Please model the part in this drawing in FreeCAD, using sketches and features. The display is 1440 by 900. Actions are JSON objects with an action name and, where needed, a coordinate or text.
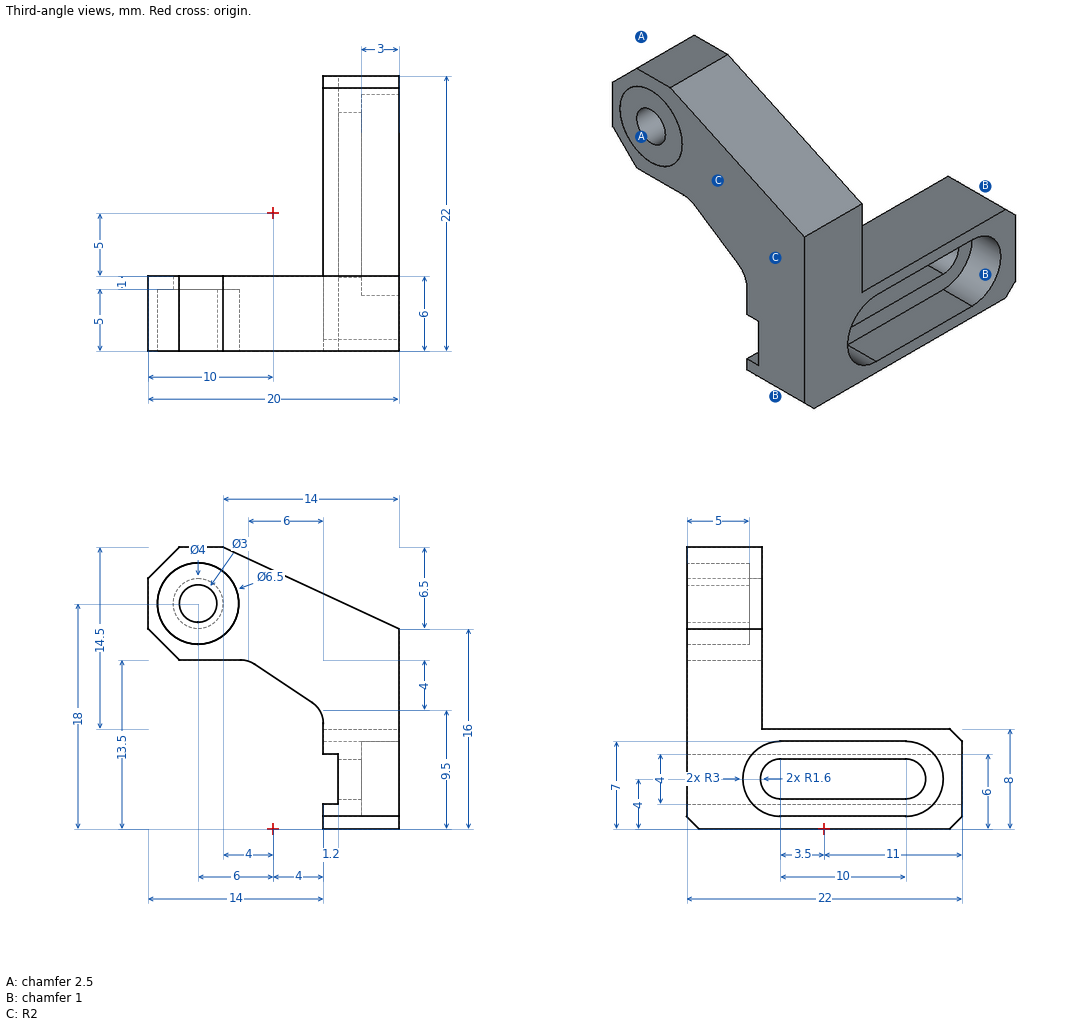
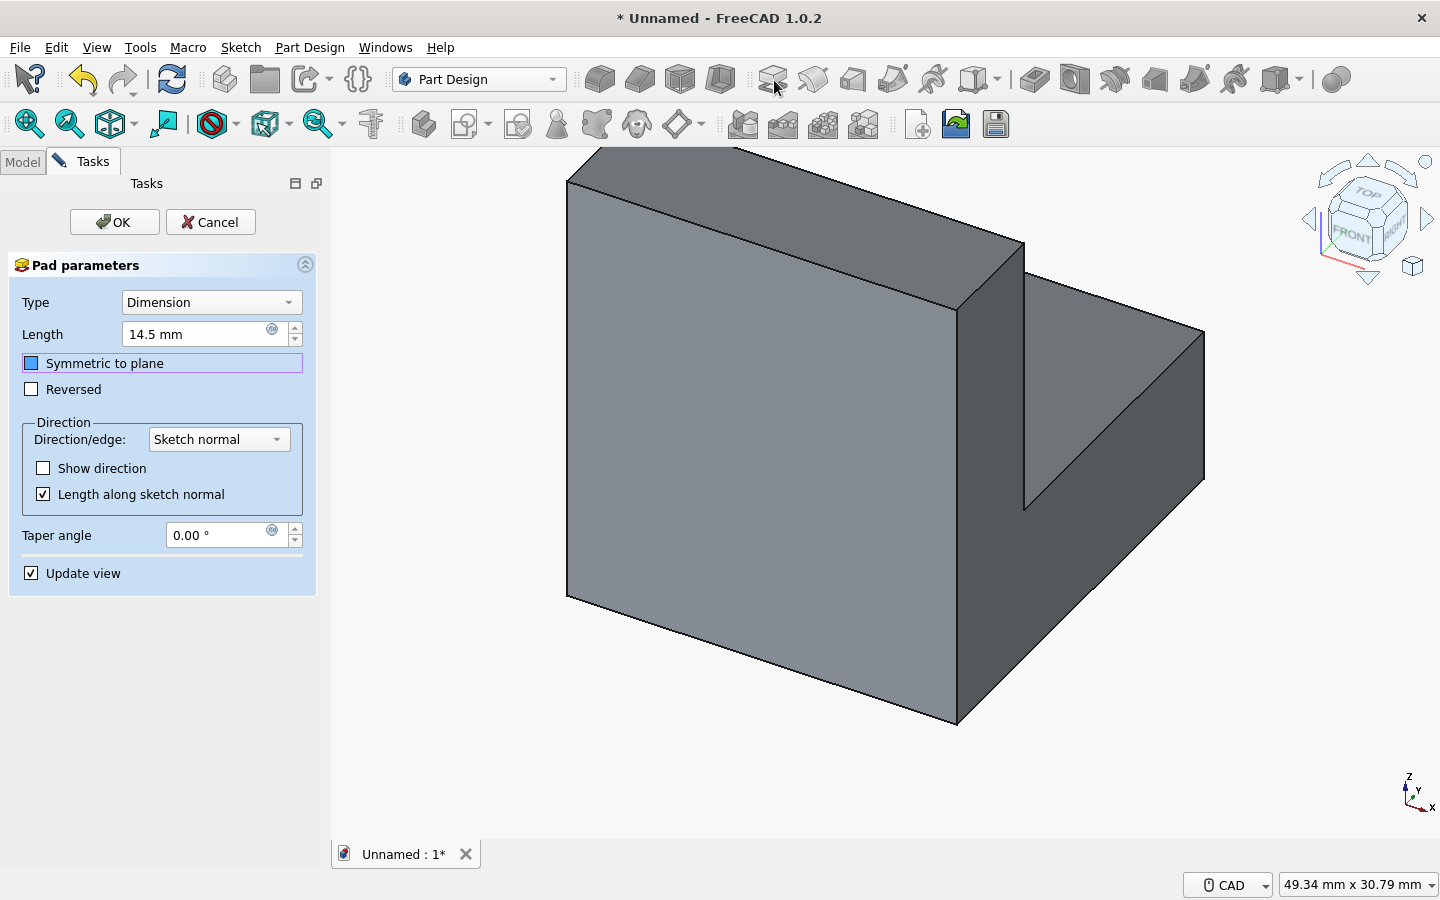
{"action": "left_click", "coordinate": [115, 222]}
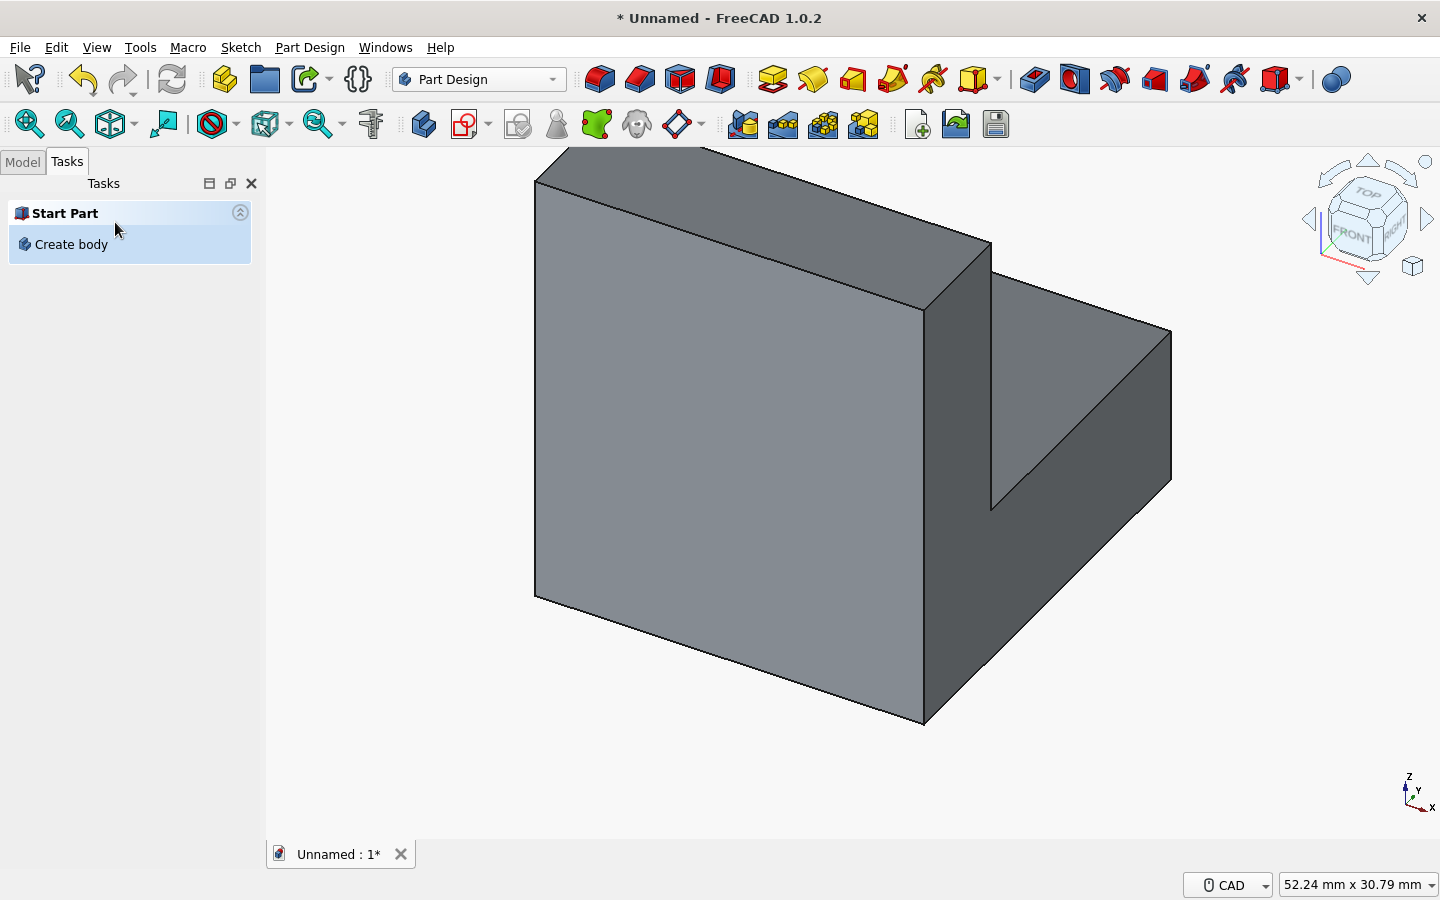
{"action": "left_click", "coordinate": [30, 124]}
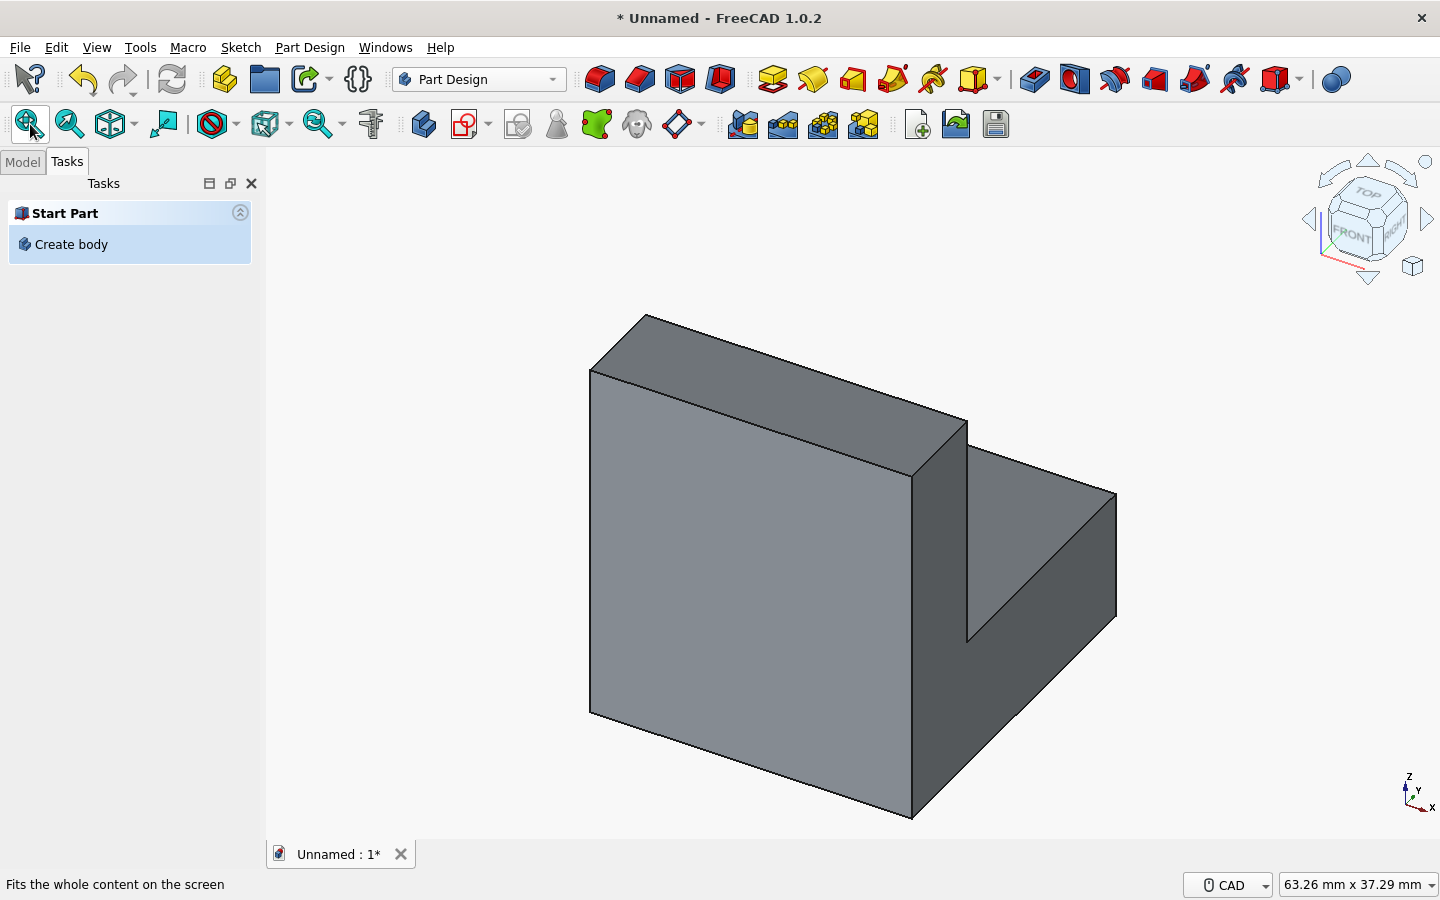
{"action": "left_click", "coordinate": [751, 593]}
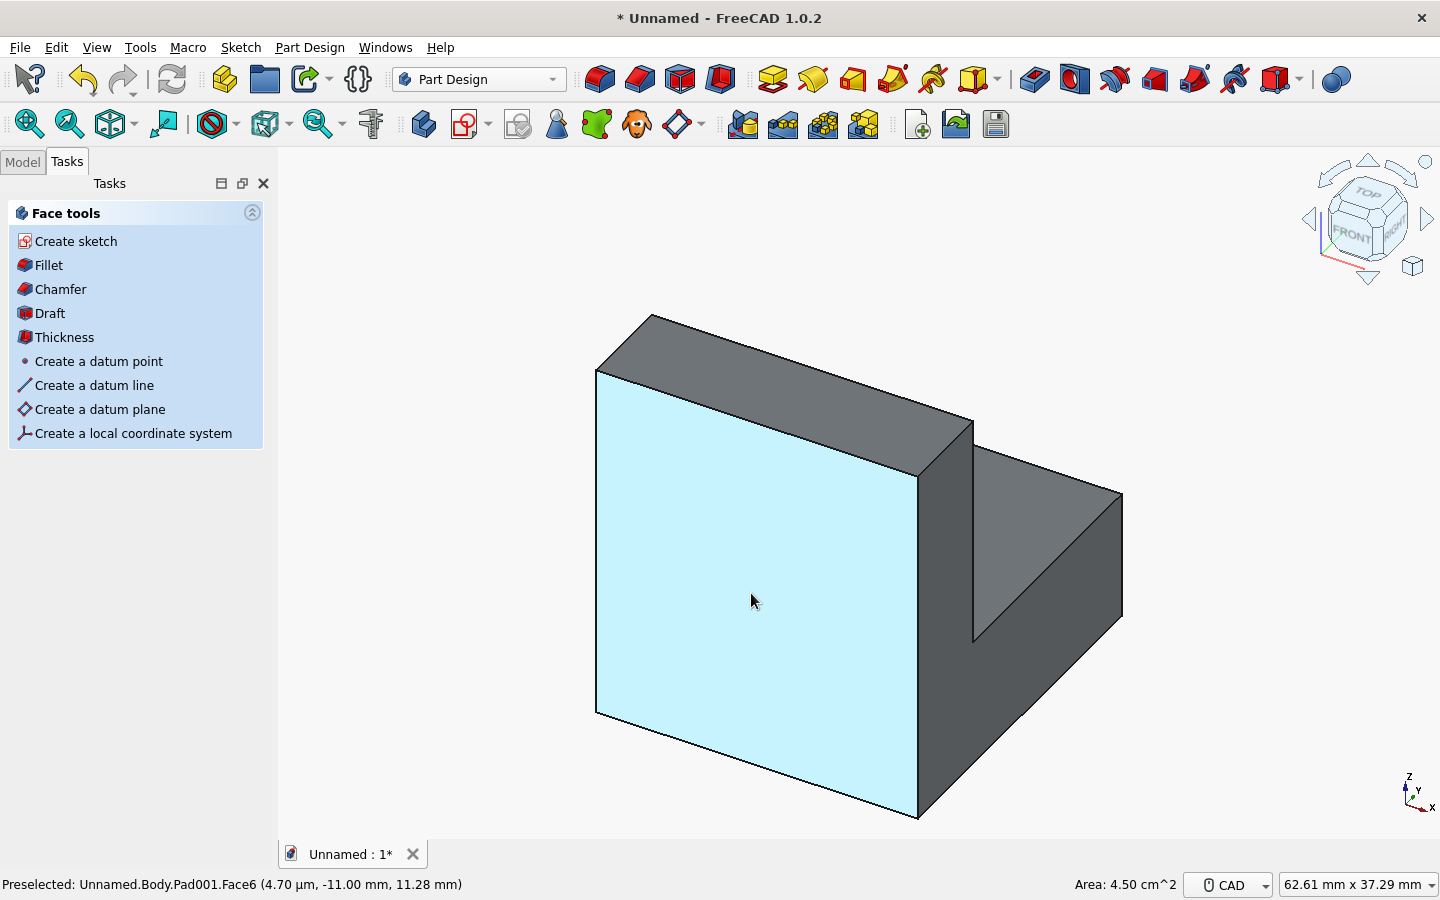
{"action": "left_click", "coordinate": [464, 124]}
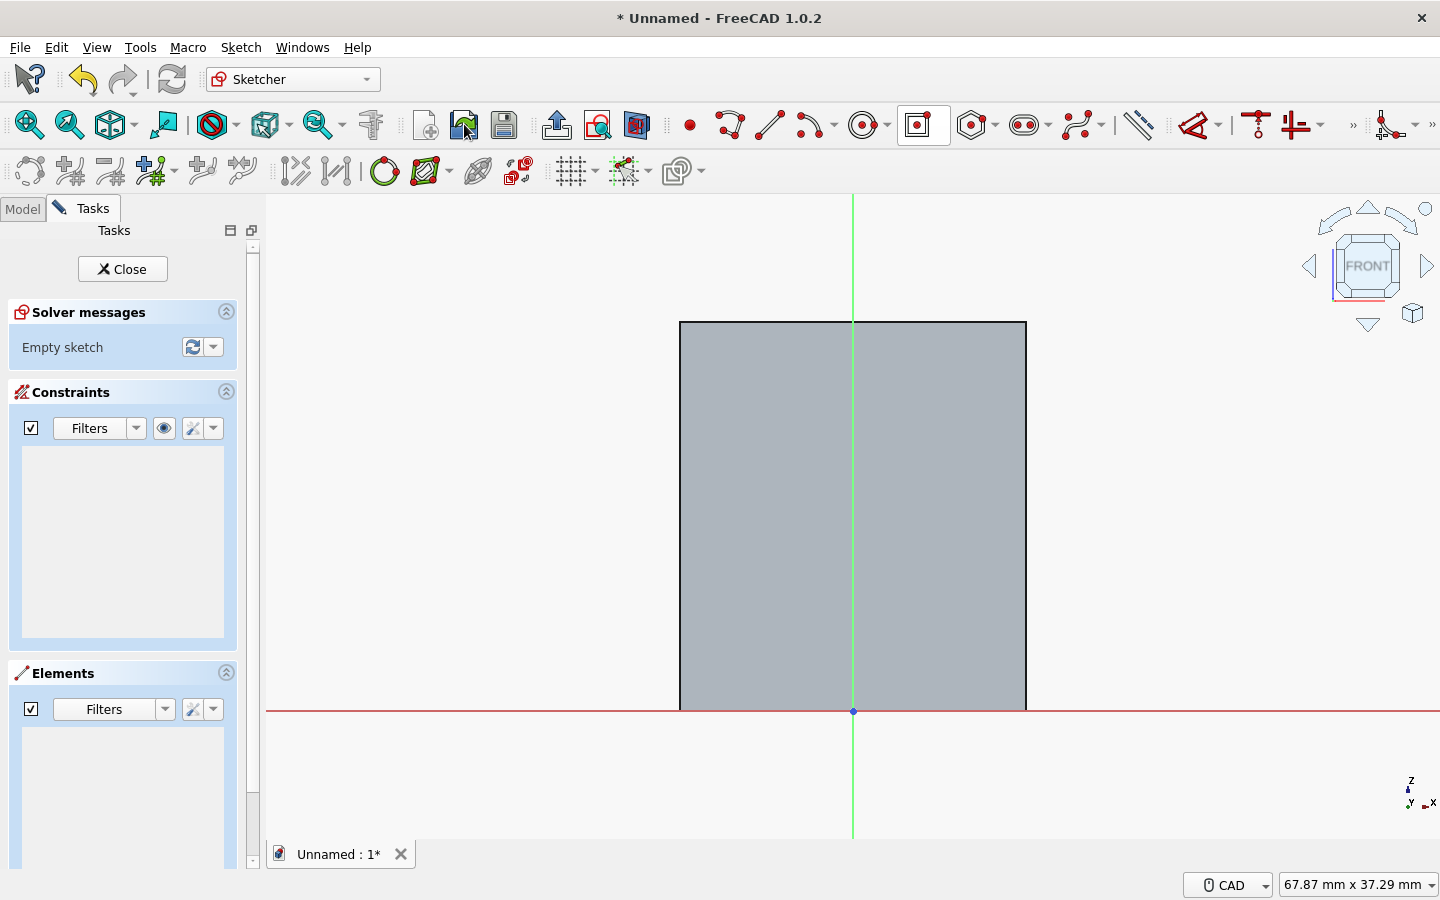
{"action": "scroll", "coordinate": [738, 362], "scroll_direction": "up", "scroll_amount": 7}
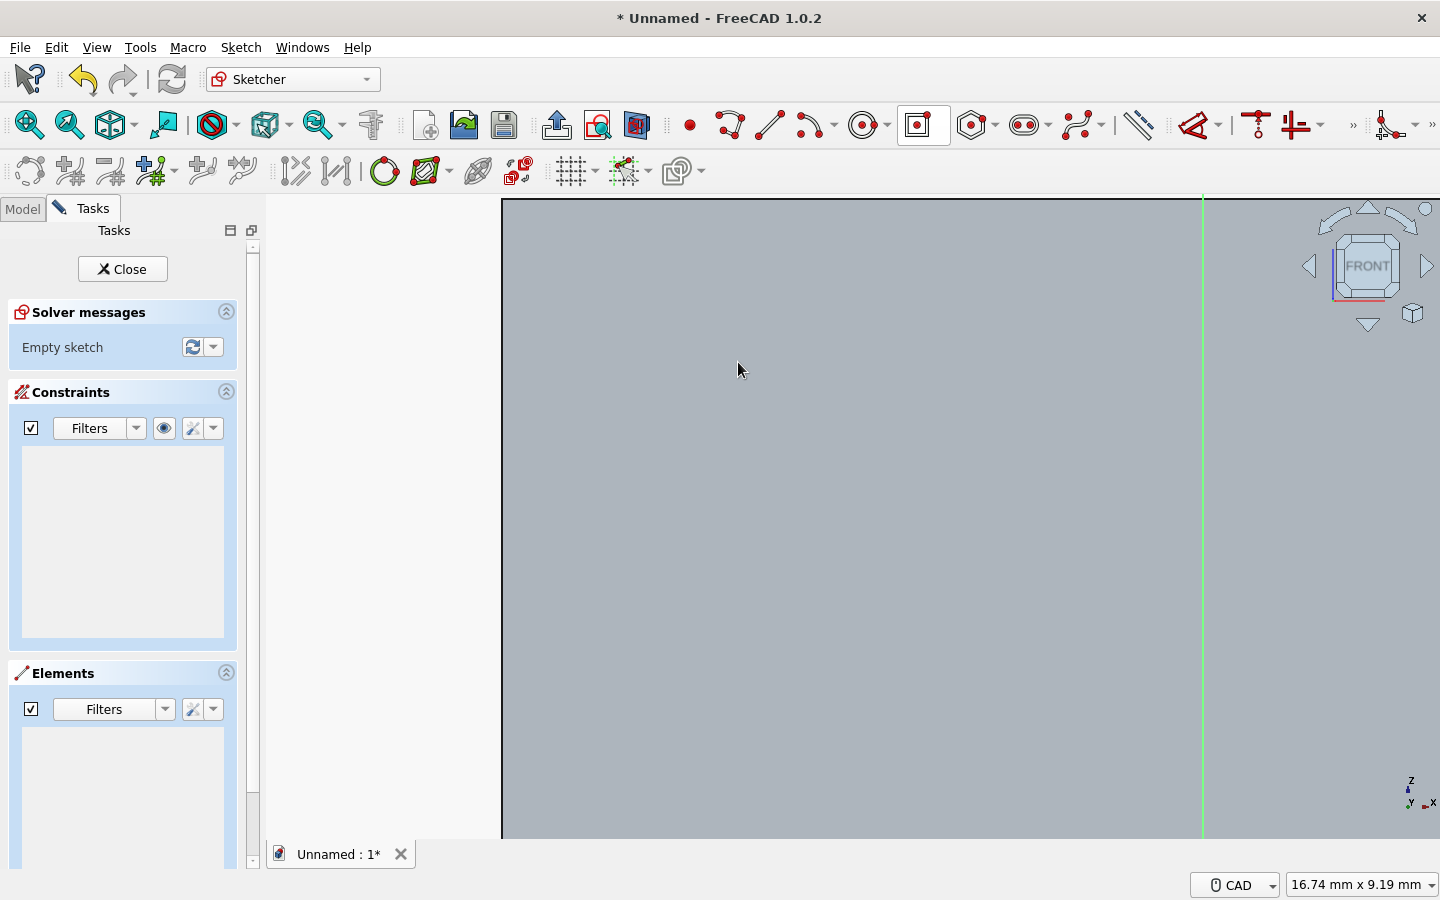
{"action": "left_click", "coordinate": [864, 126]}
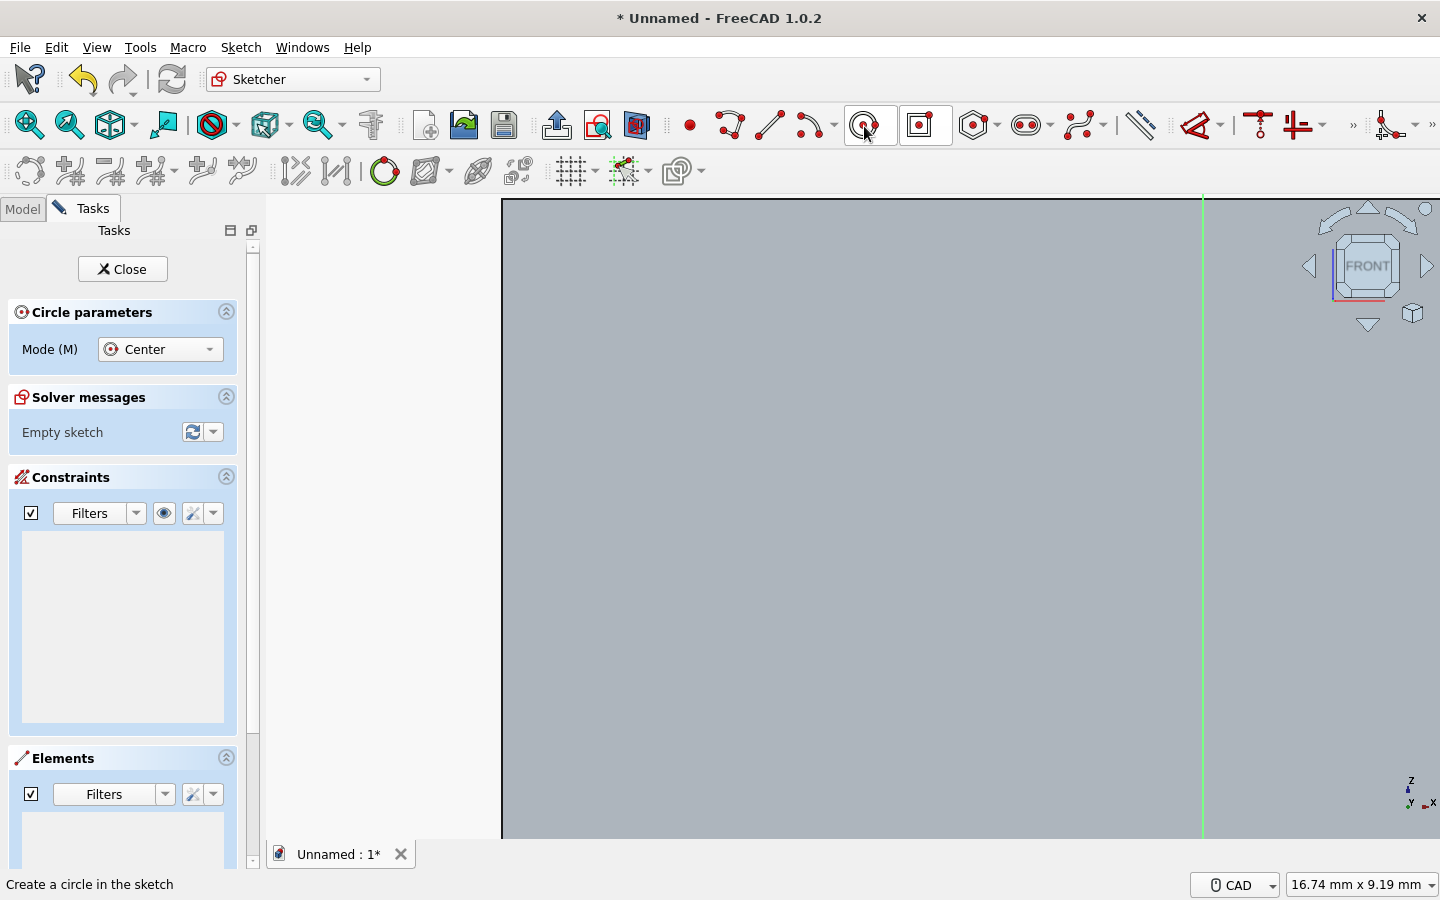
{"action": "left_click", "coordinate": [782, 514]}
{"action": "mouse_move", "coordinate": [943, 353]}